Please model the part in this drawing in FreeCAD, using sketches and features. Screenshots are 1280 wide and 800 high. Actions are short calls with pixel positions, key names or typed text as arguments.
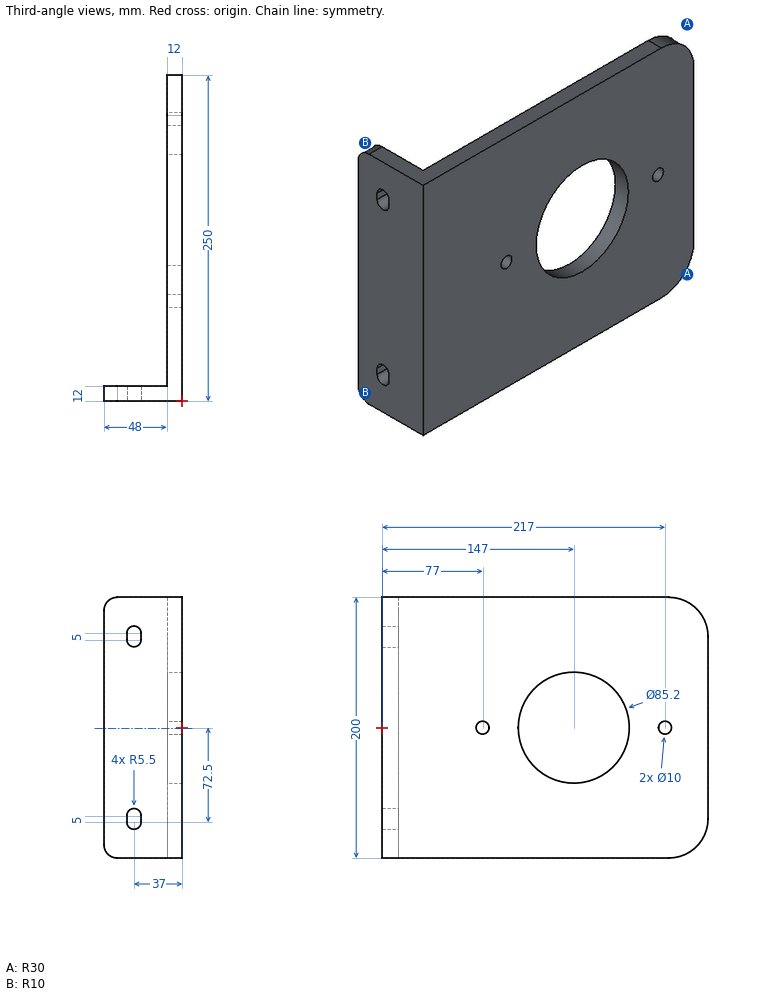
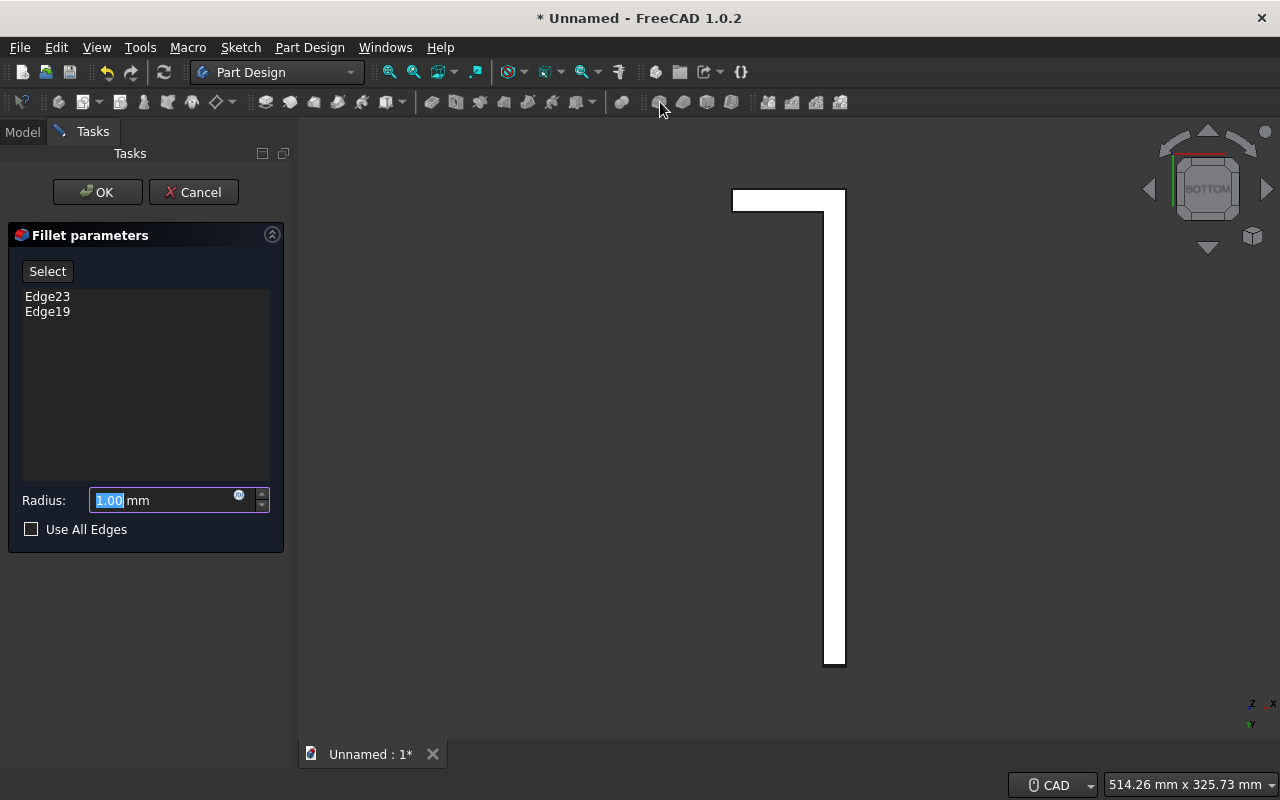
text(30)
key(Tab)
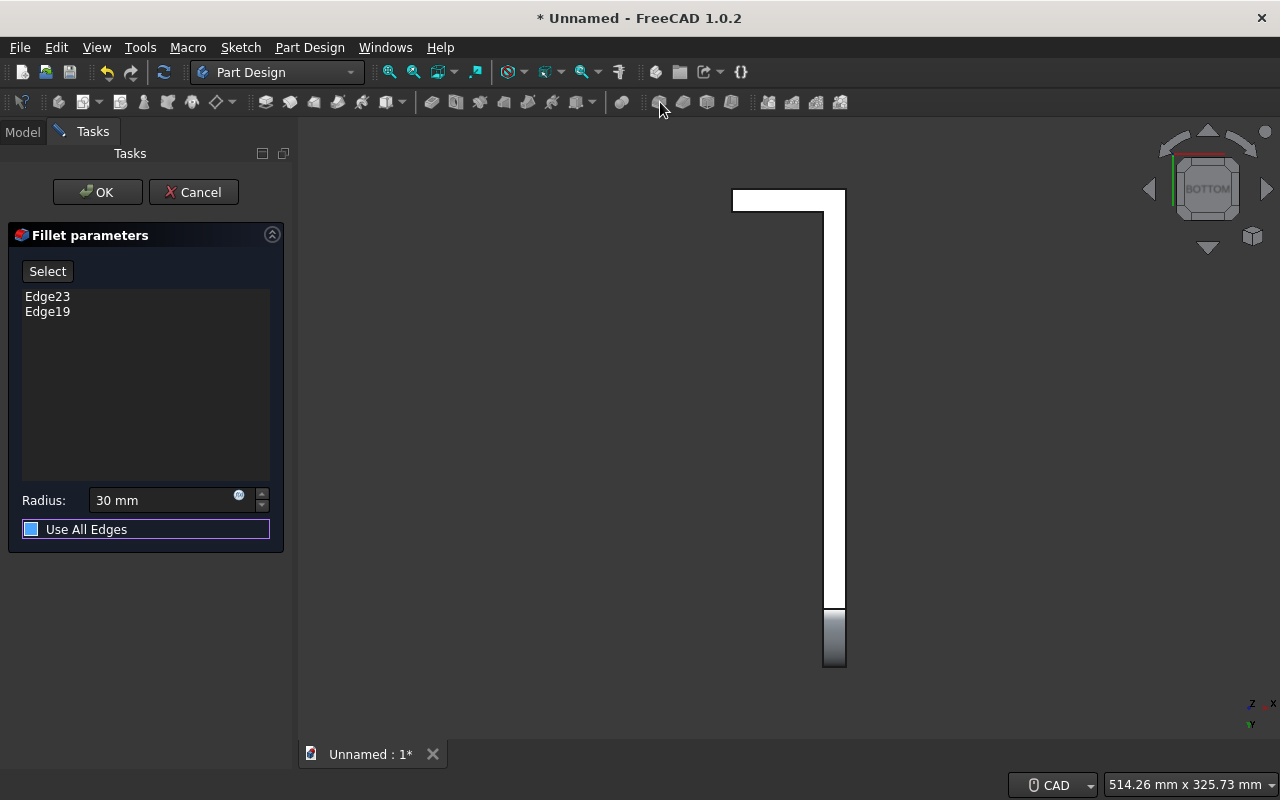
click(98, 192)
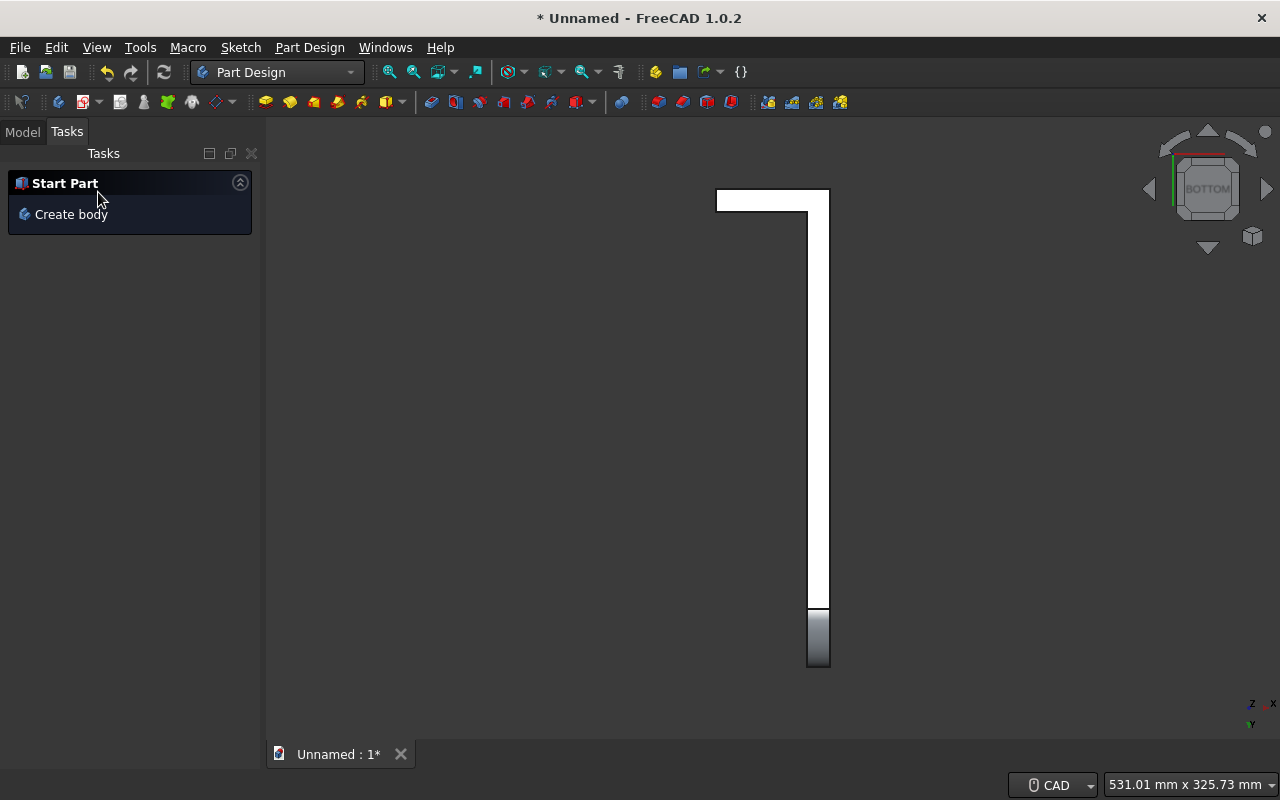
click(716, 200)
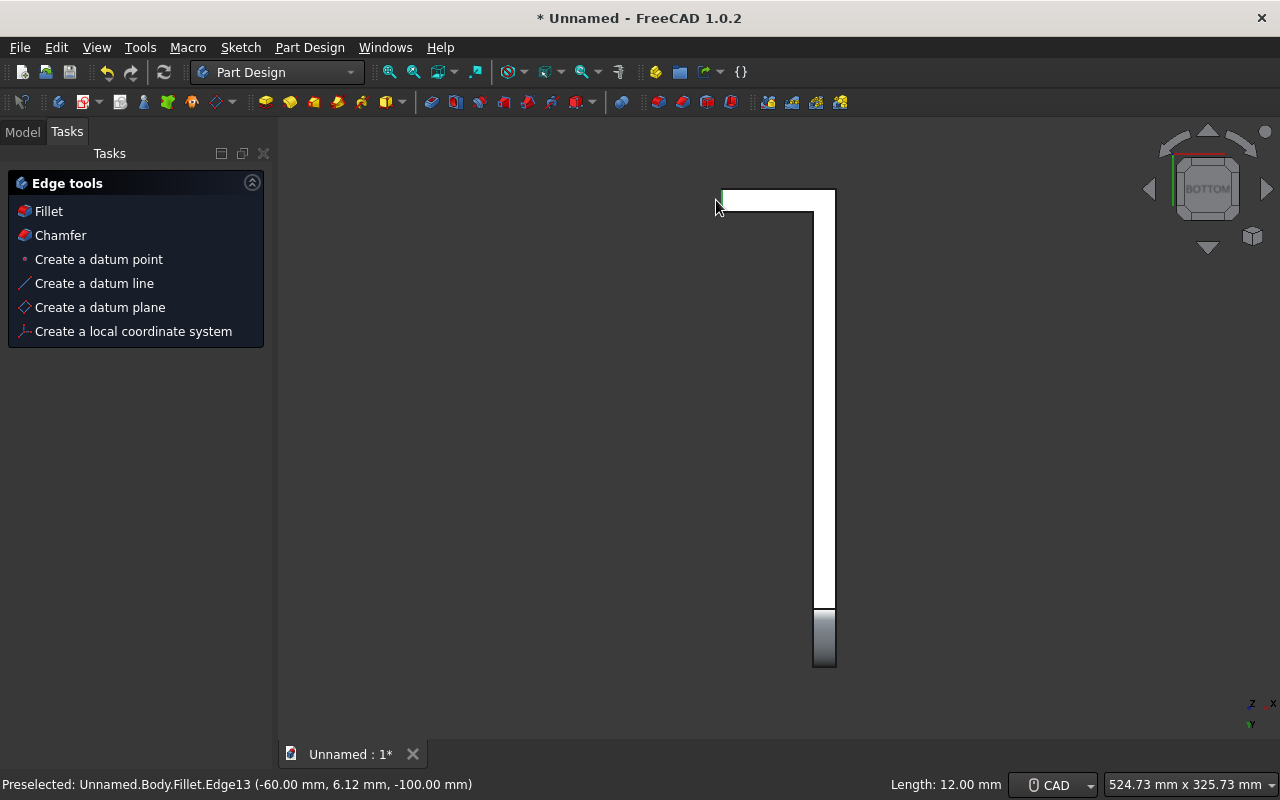
key(0)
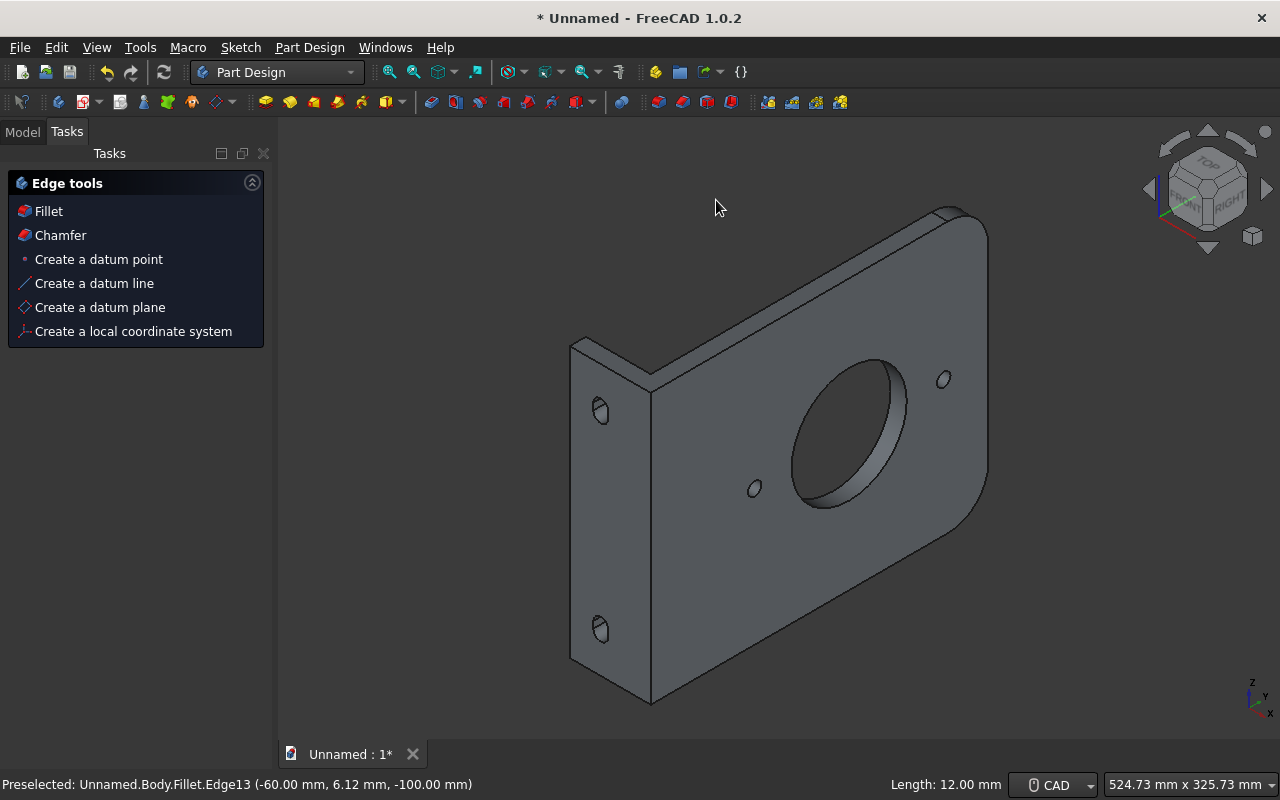
key(2)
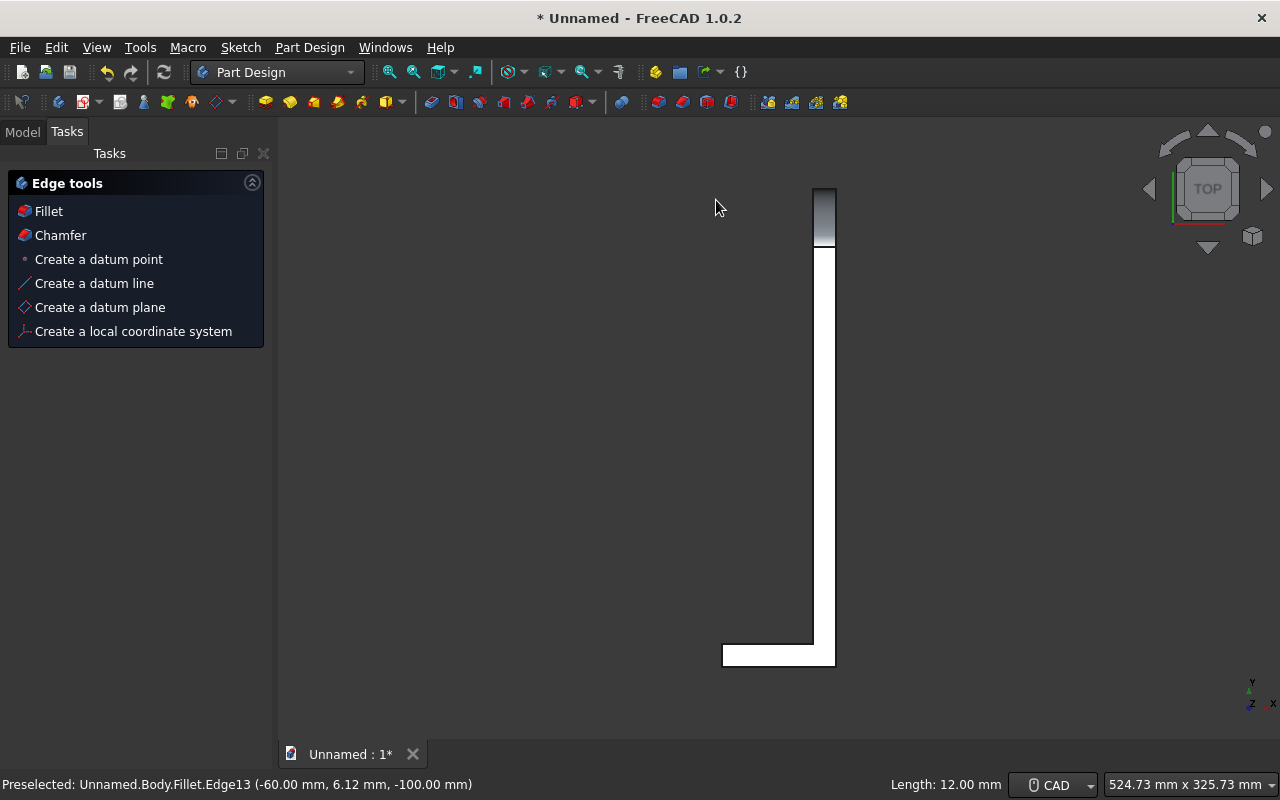
click(722, 654, ctrl)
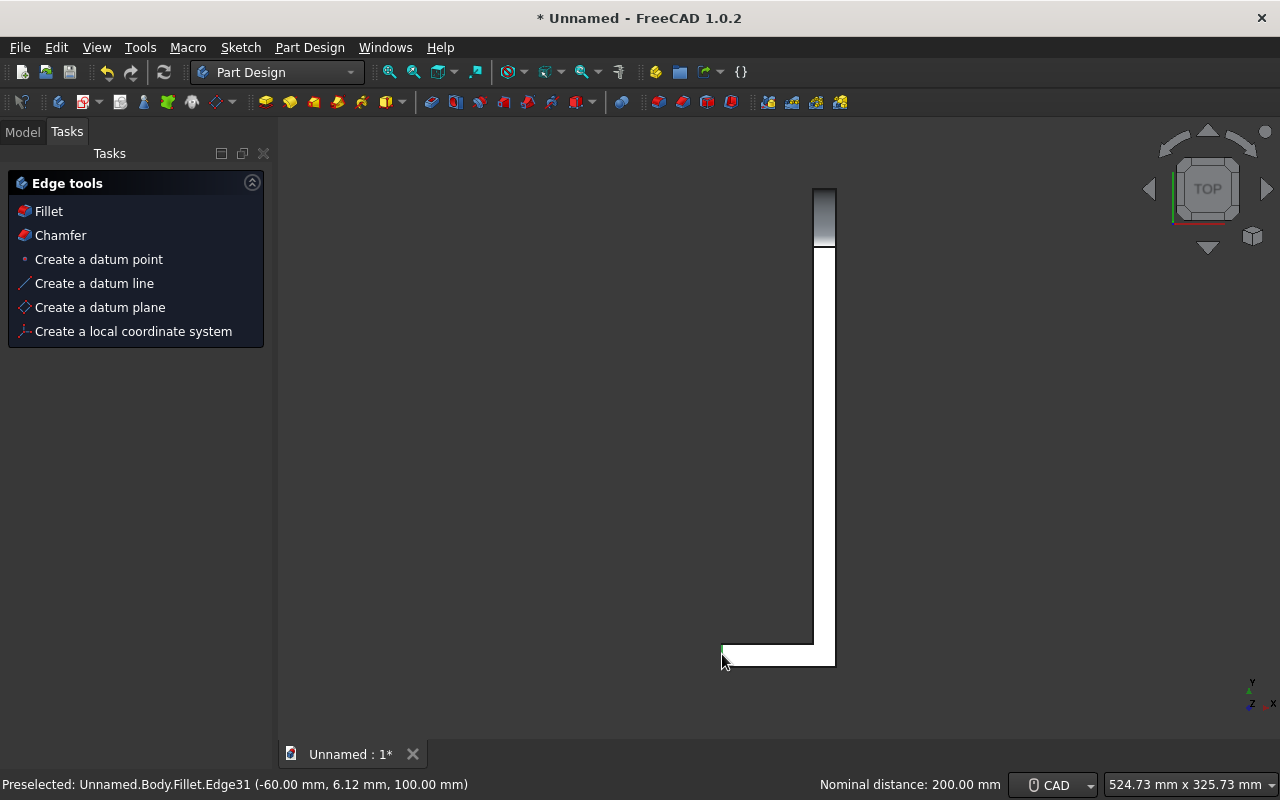
click(660, 102)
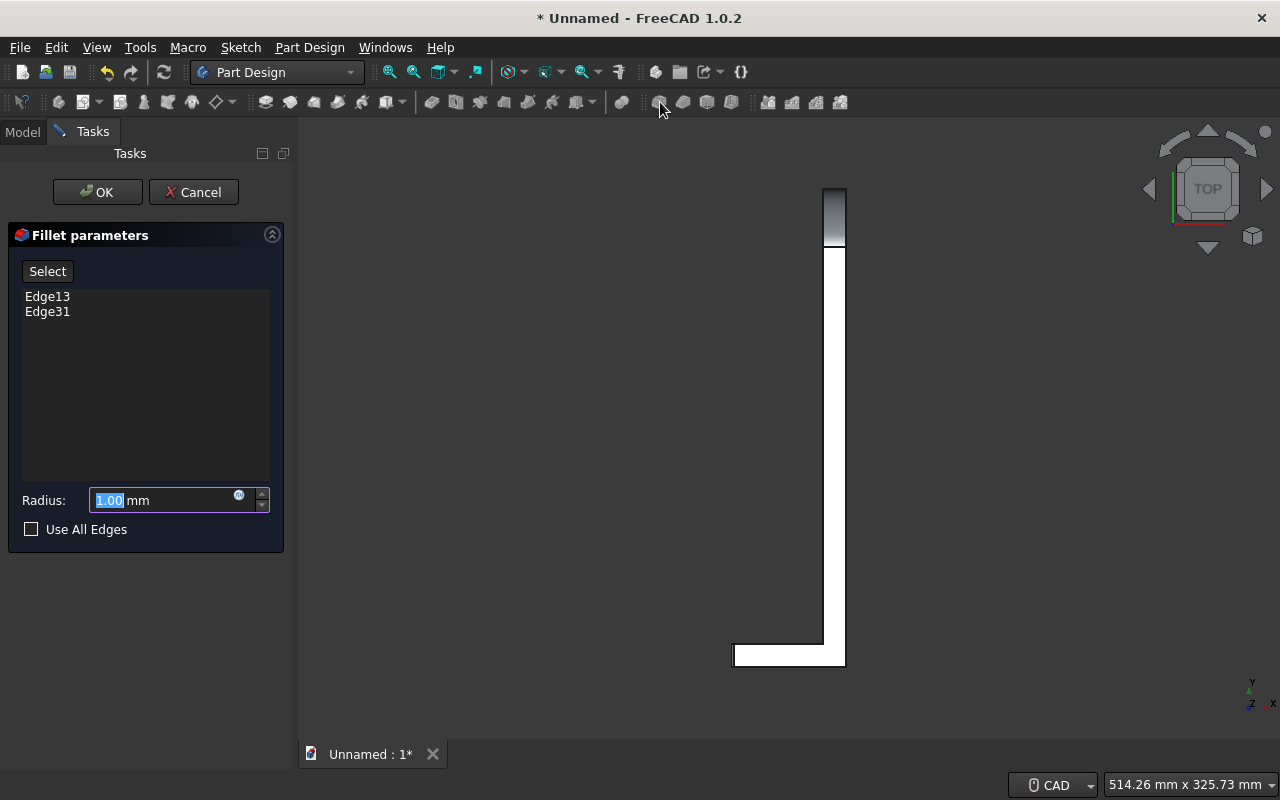
text(10)
key(Tab)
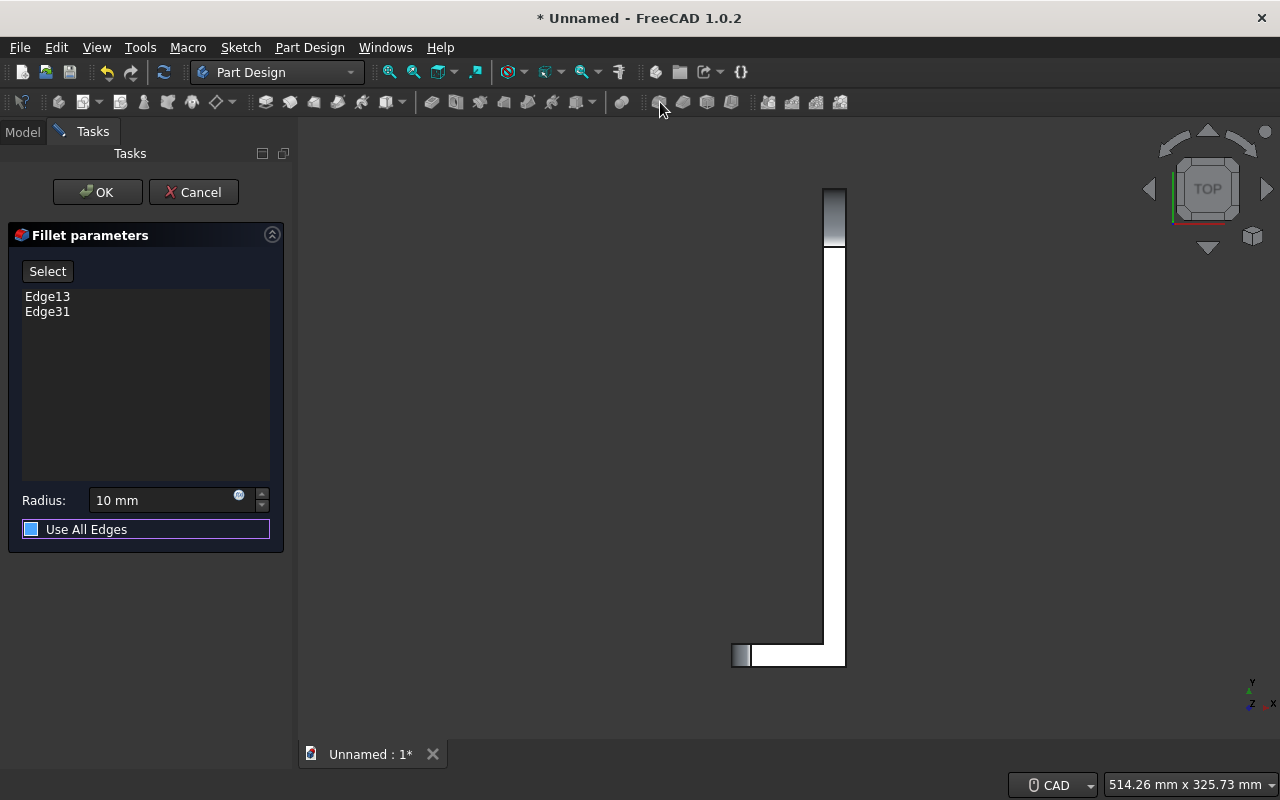
click(98, 192)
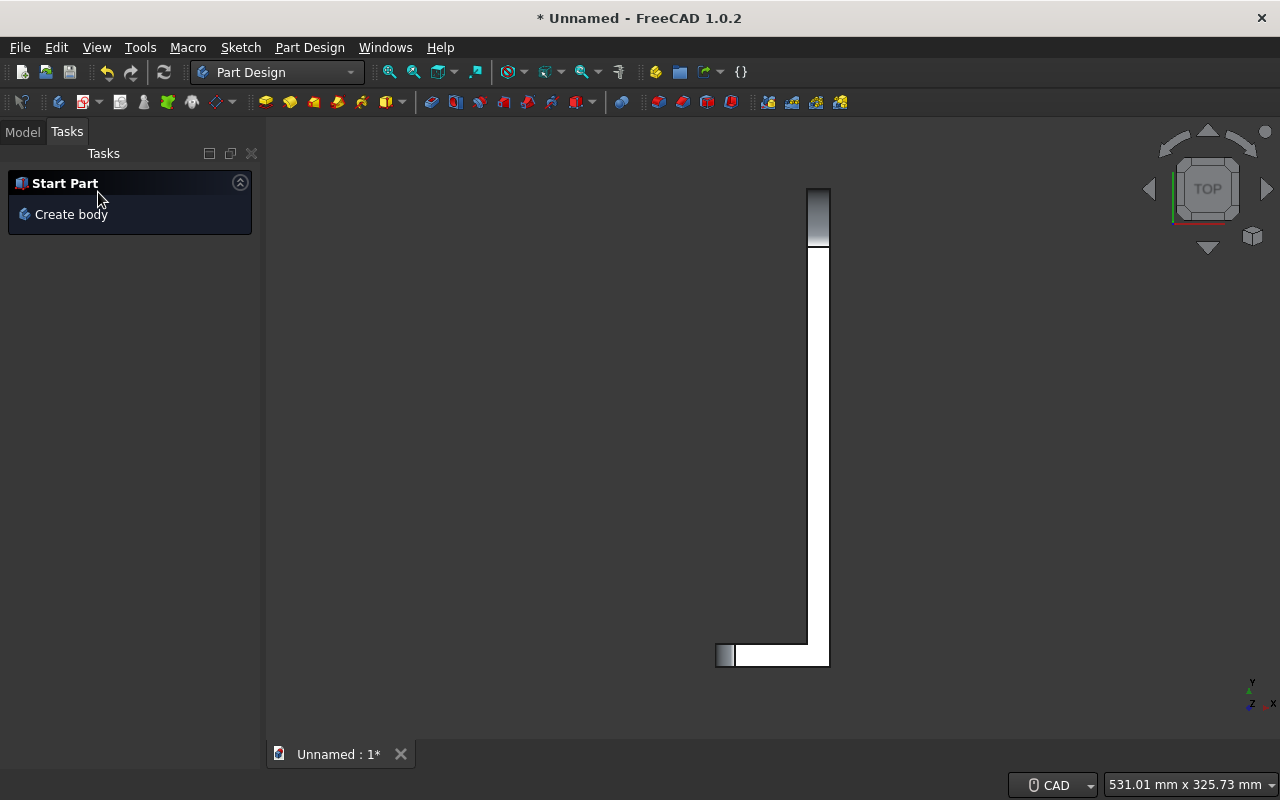
key(0)